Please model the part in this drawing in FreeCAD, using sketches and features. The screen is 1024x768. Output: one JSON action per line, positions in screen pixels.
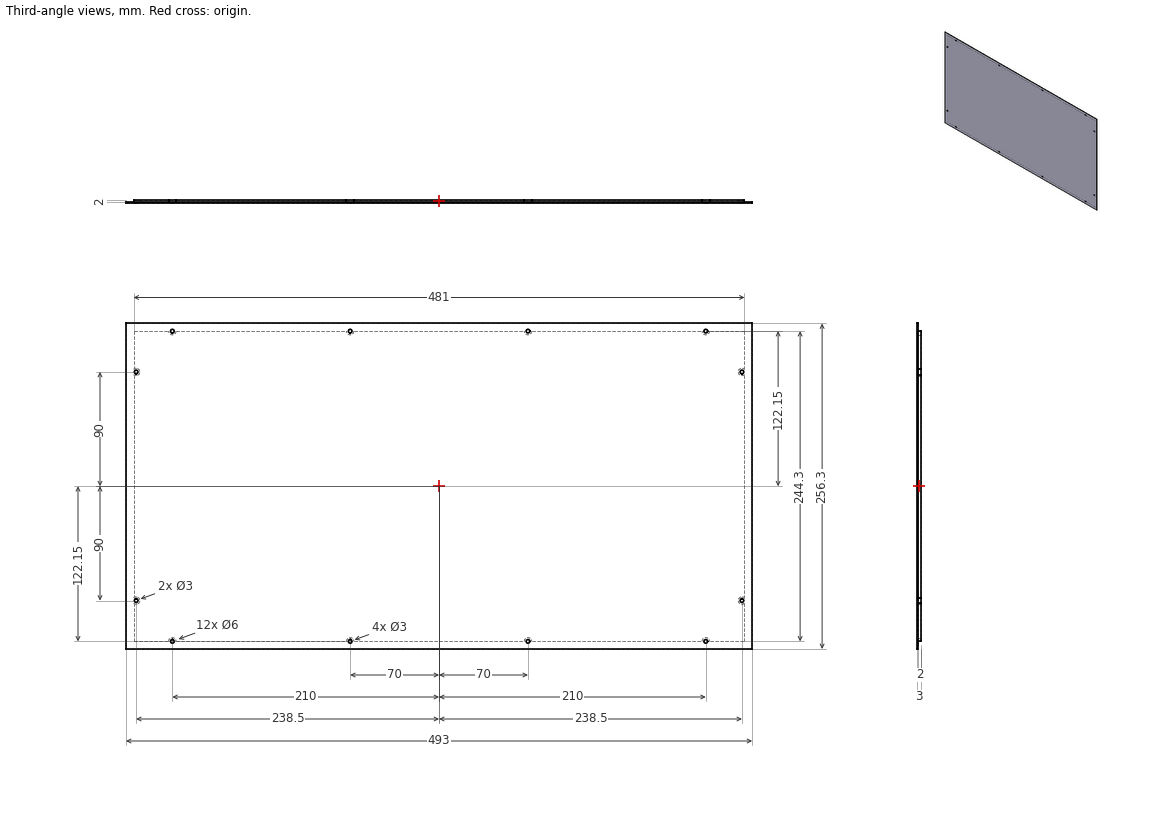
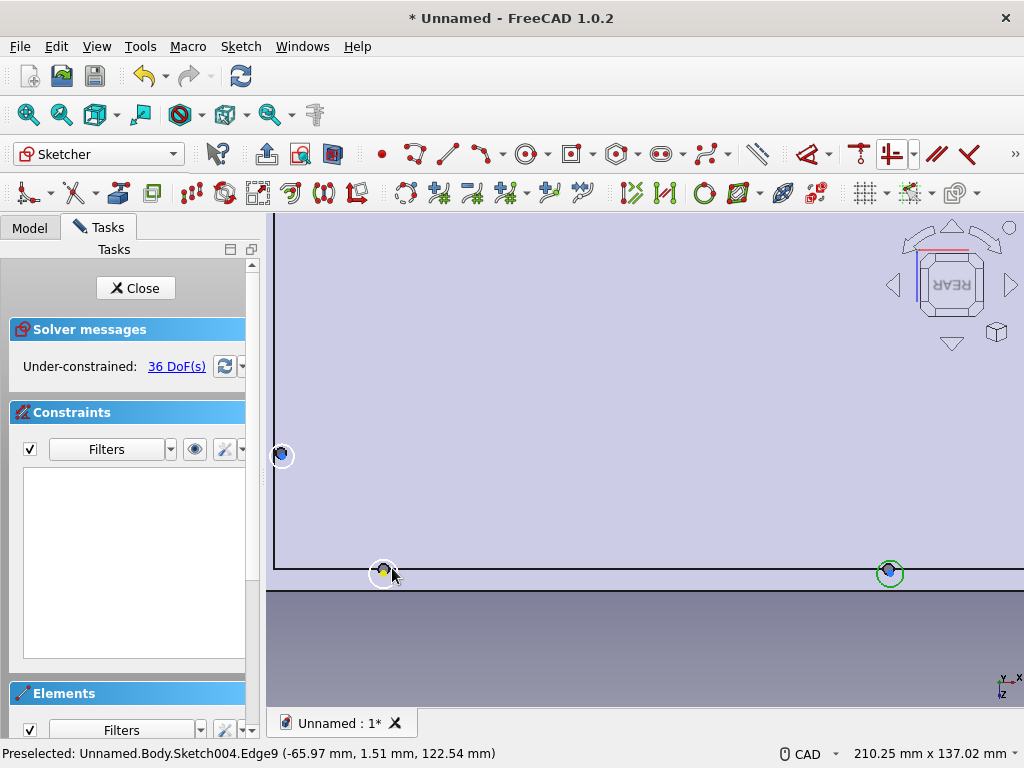
{"action": "left_click", "coordinate": [393, 564]}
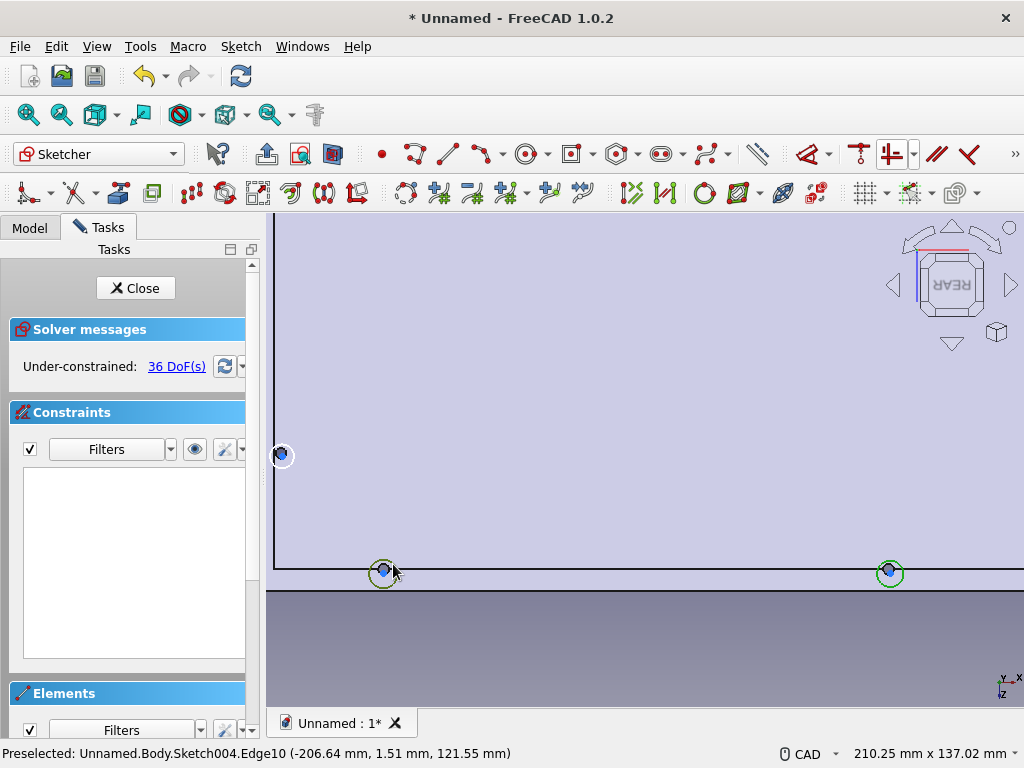
{"action": "scroll", "coordinate": [392, 568], "scroll_direction": "down", "scroll_amount": 7}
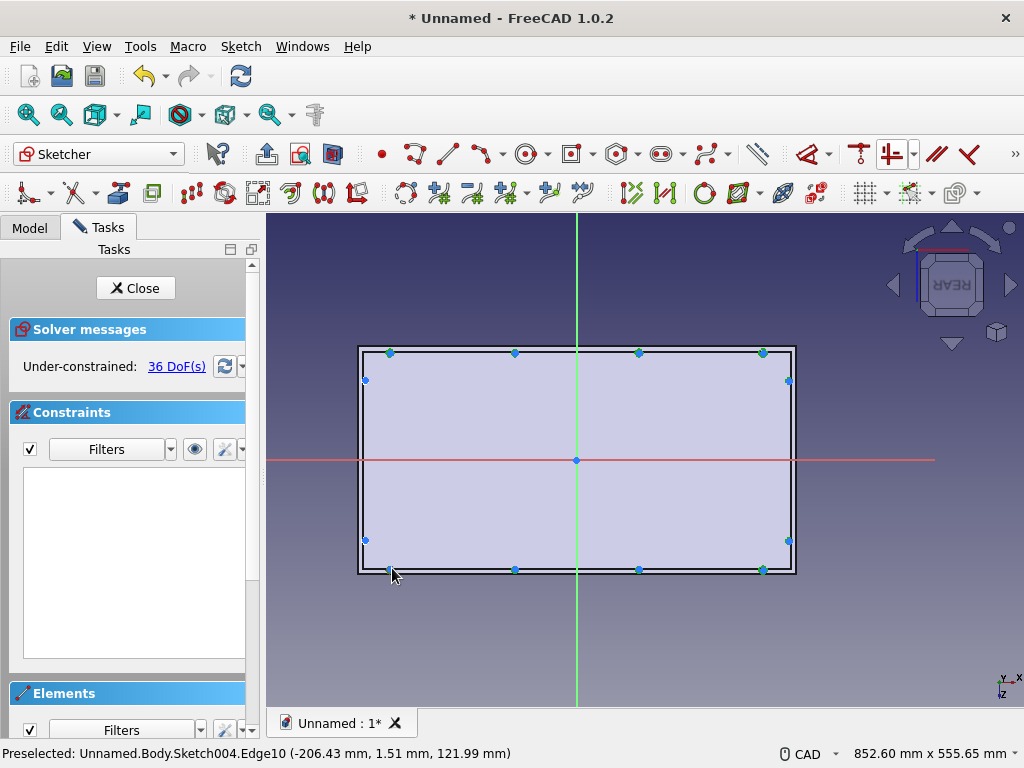
{"action": "scroll", "coordinate": [367, 539], "scroll_direction": "up", "scroll_amount": 8}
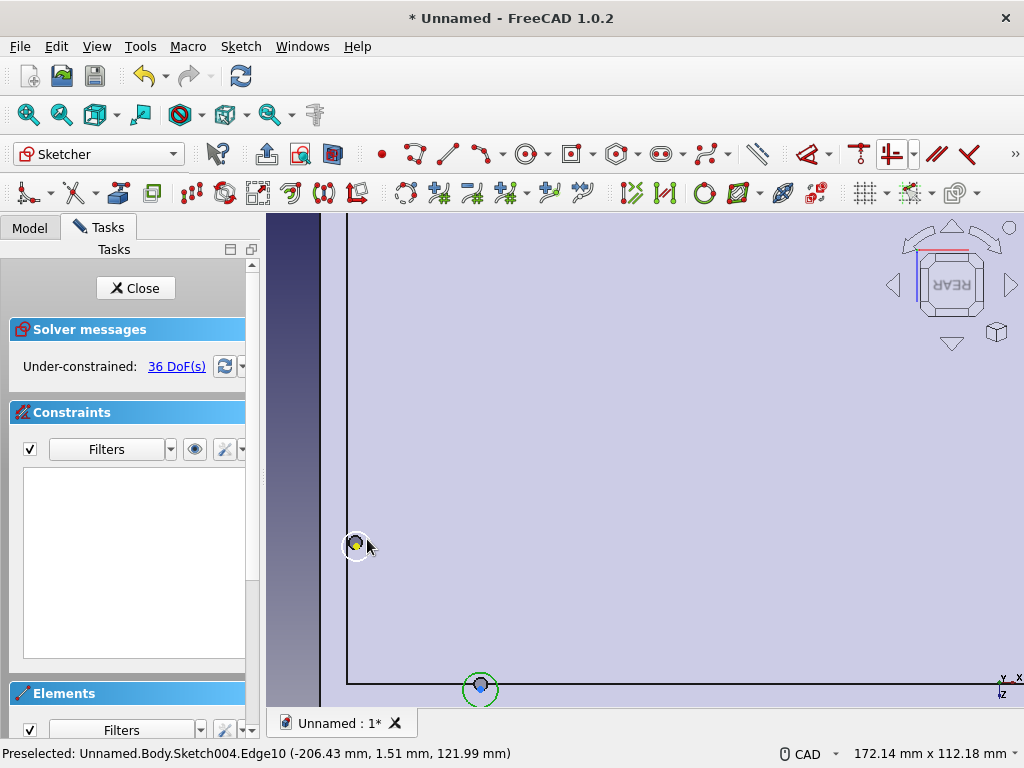
{"action": "left_click", "coordinate": [367, 536]}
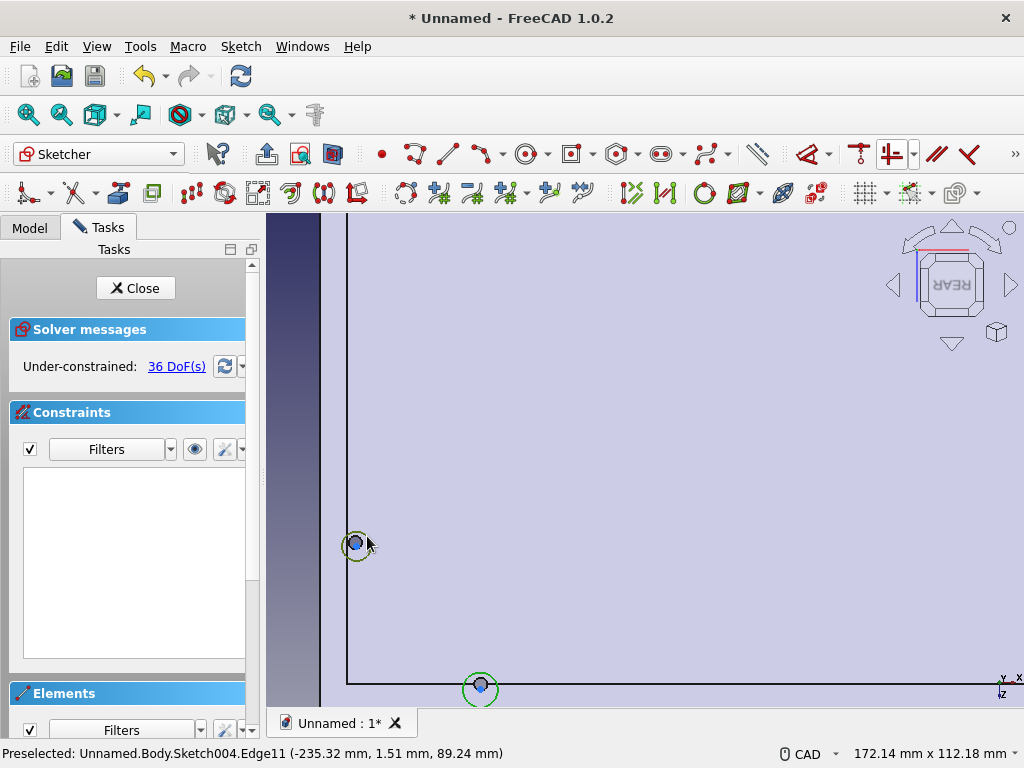
{"action": "scroll", "coordinate": [367, 539], "scroll_direction": "down", "scroll_amount": 8}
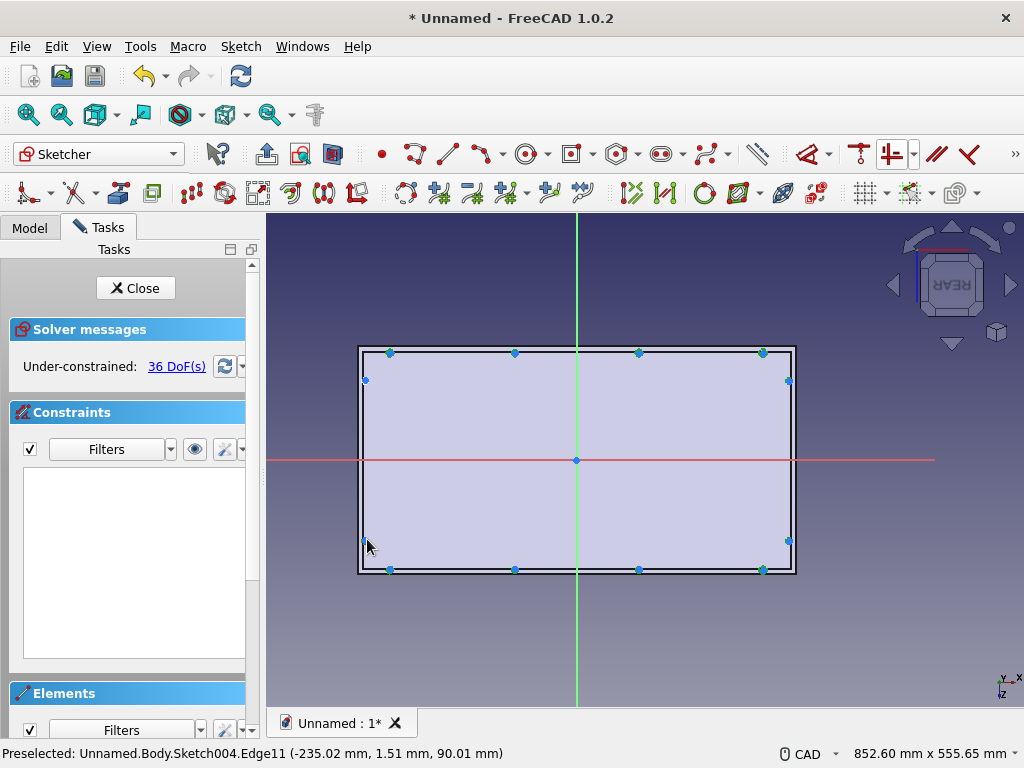
{"action": "scroll", "coordinate": [367, 379], "scroll_direction": "up", "scroll_amount": 8}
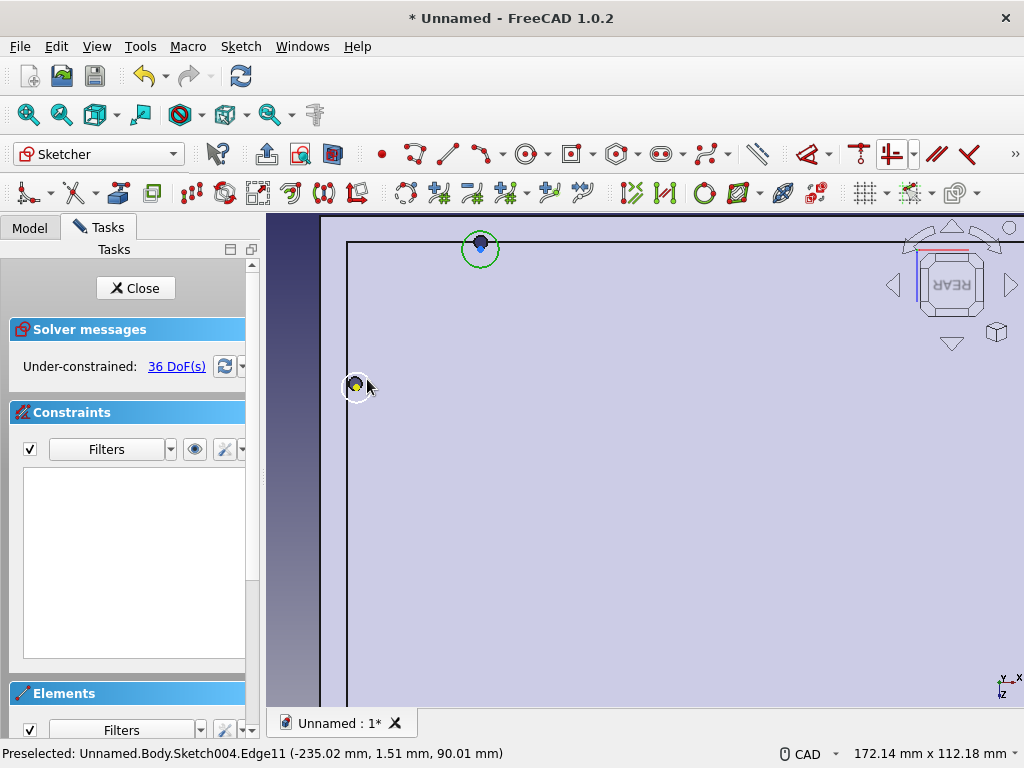
{"action": "left_click", "coordinate": [367, 377]}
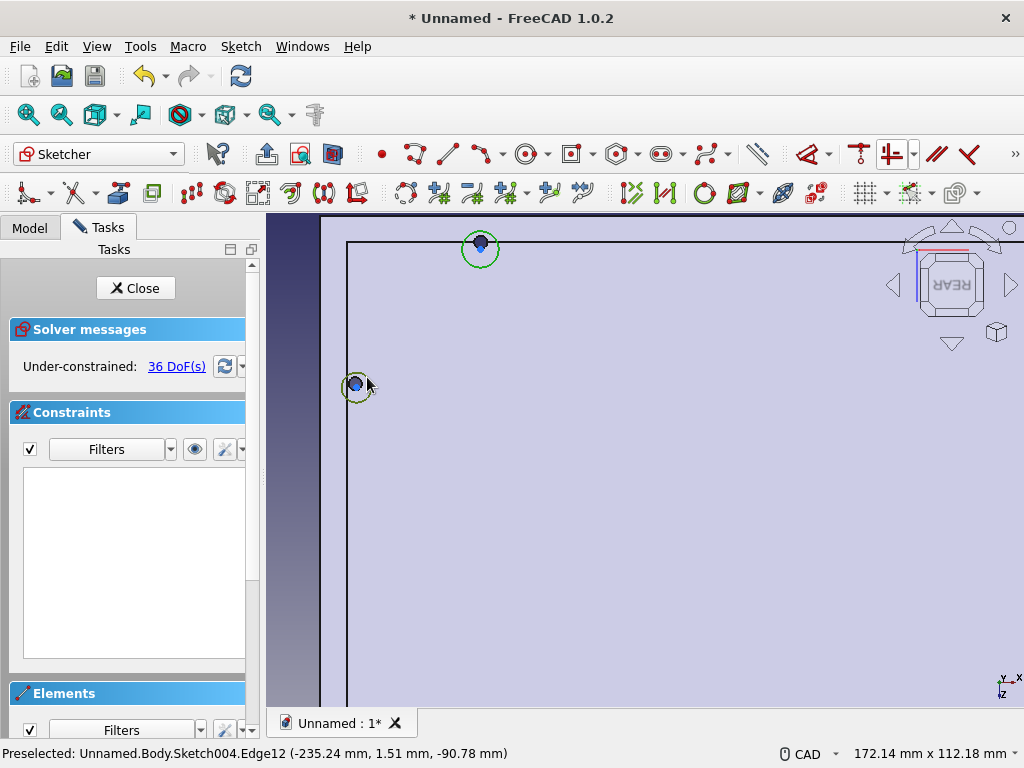
{"action": "key", "text": "e"}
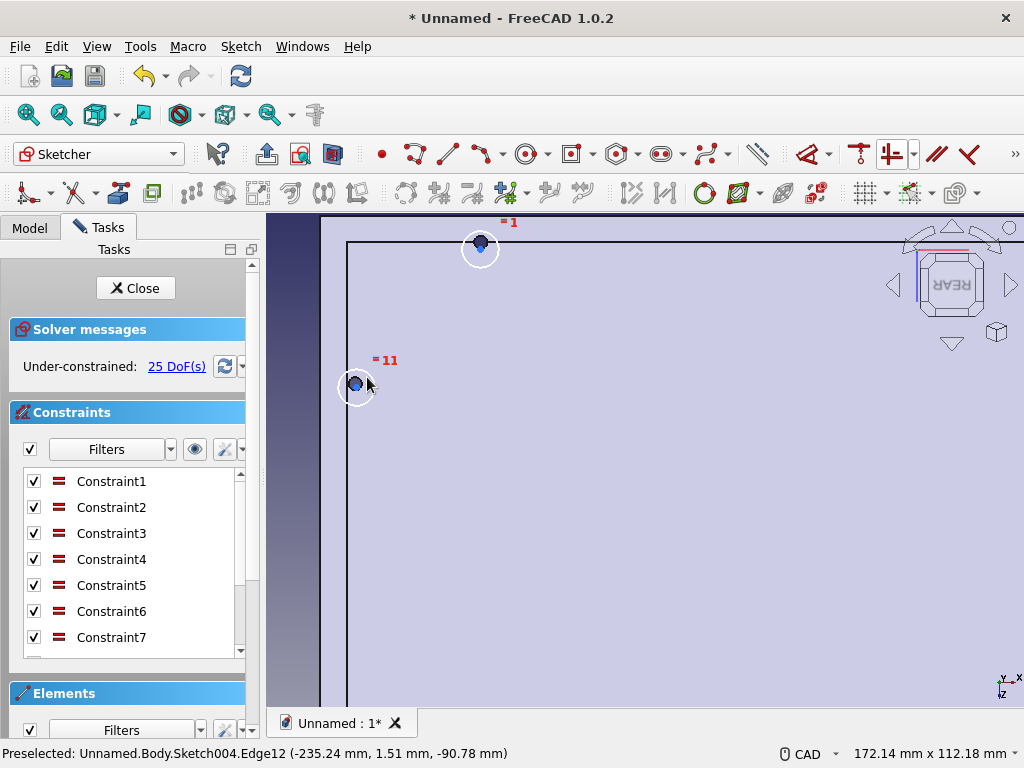
{"action": "scroll", "coordinate": [367, 379], "scroll_direction": "down", "scroll_amount": 8}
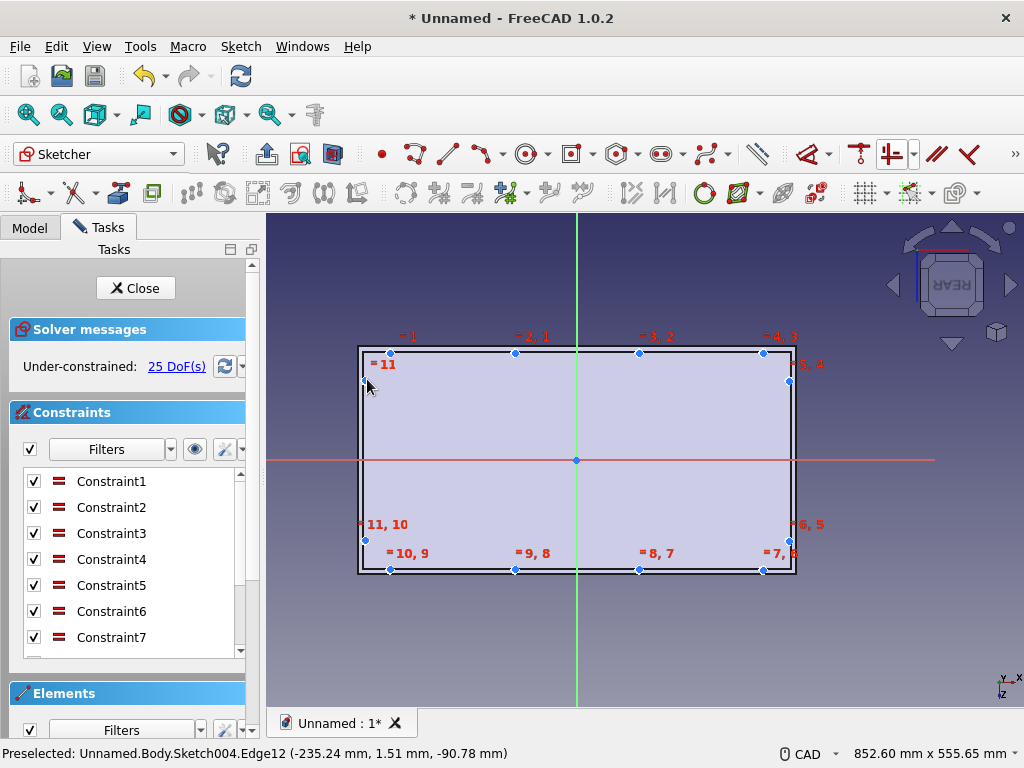
{"action": "left_click", "coordinate": [390, 353]}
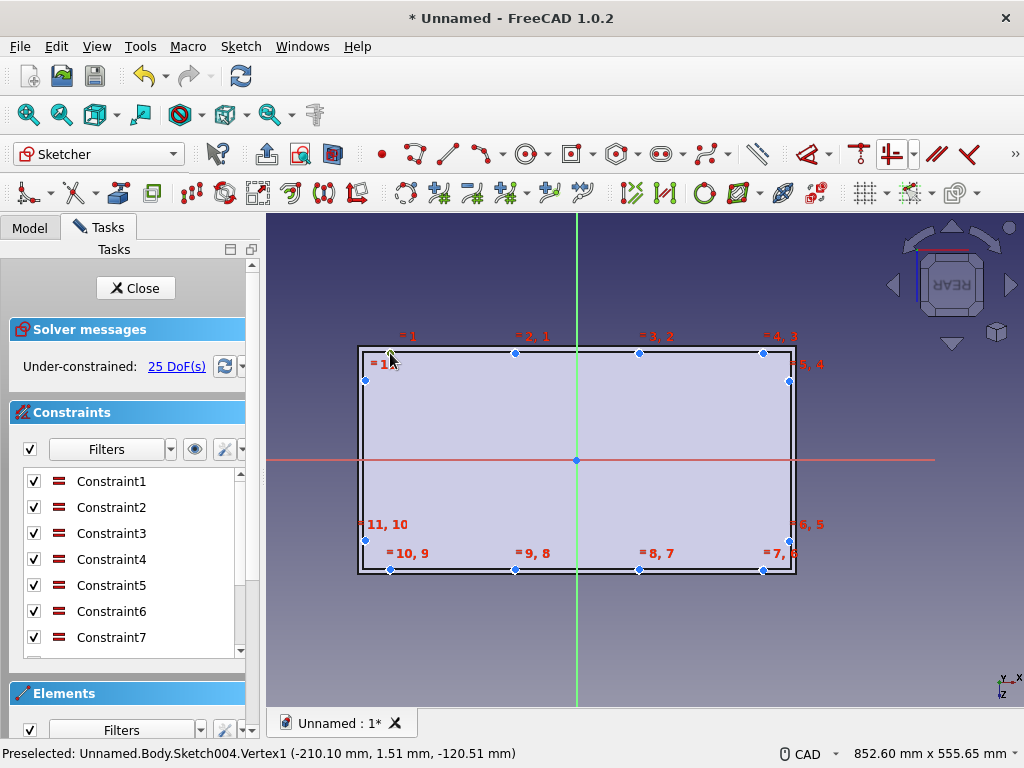
{"action": "left_click", "coordinate": [515, 353]}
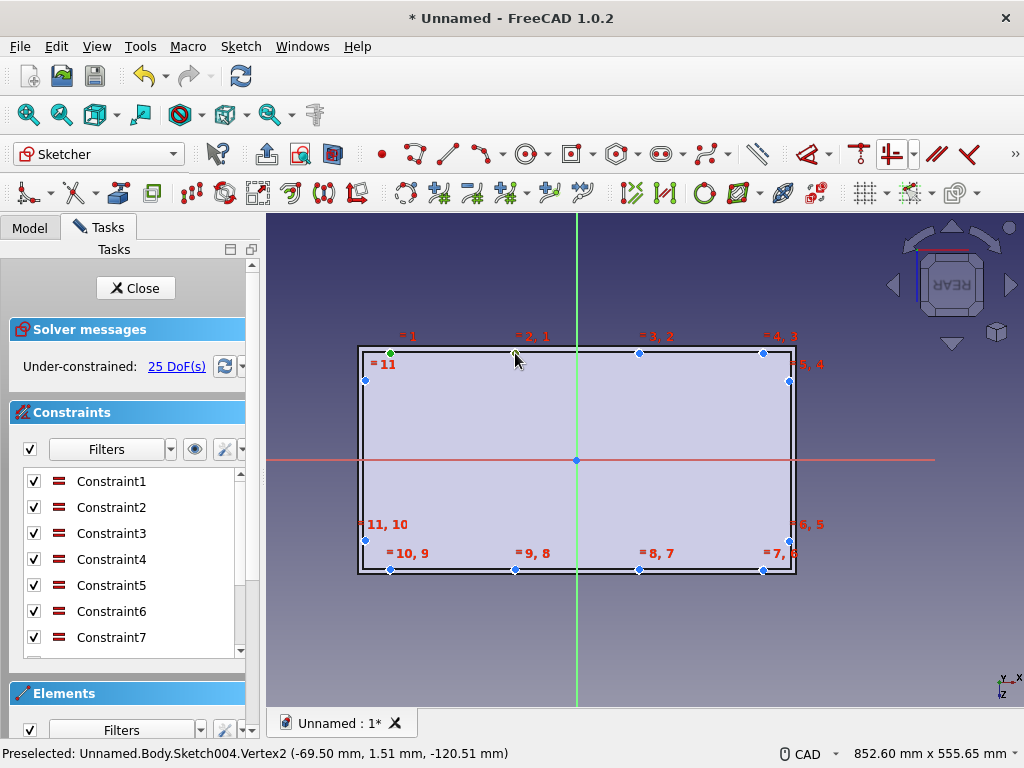
{"action": "key", "text": "h"}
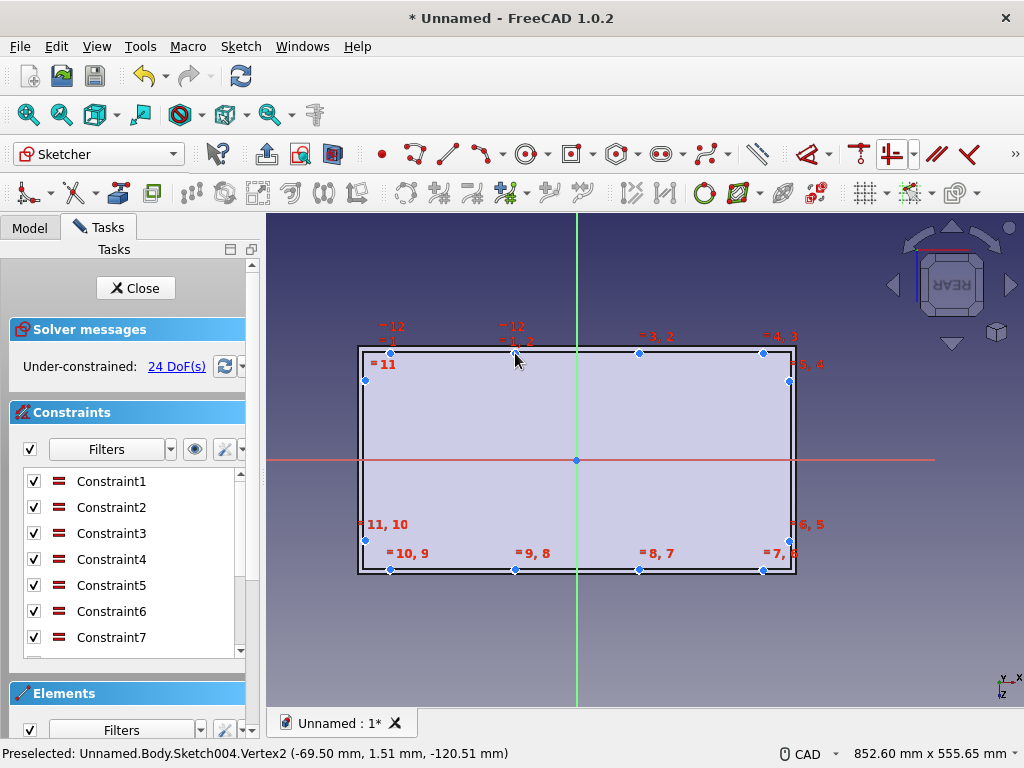
{"action": "left_click", "coordinate": [515, 353]}